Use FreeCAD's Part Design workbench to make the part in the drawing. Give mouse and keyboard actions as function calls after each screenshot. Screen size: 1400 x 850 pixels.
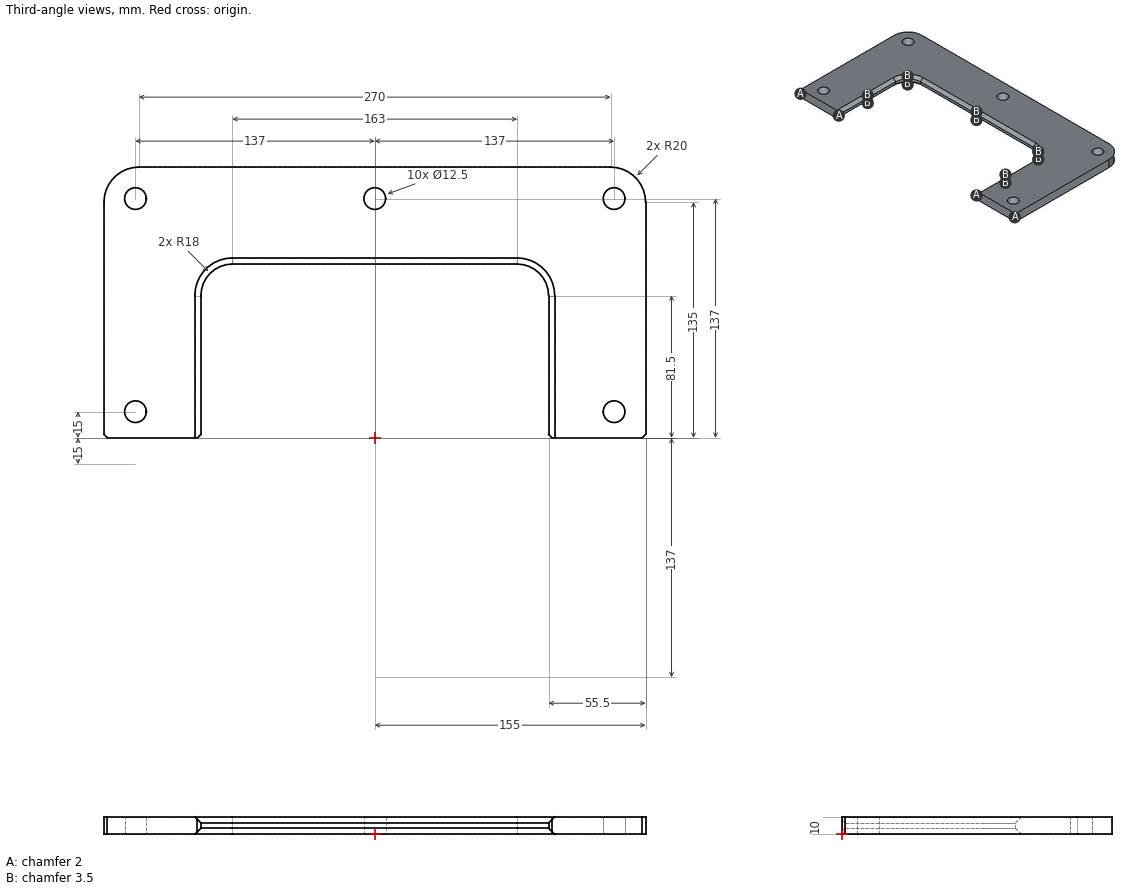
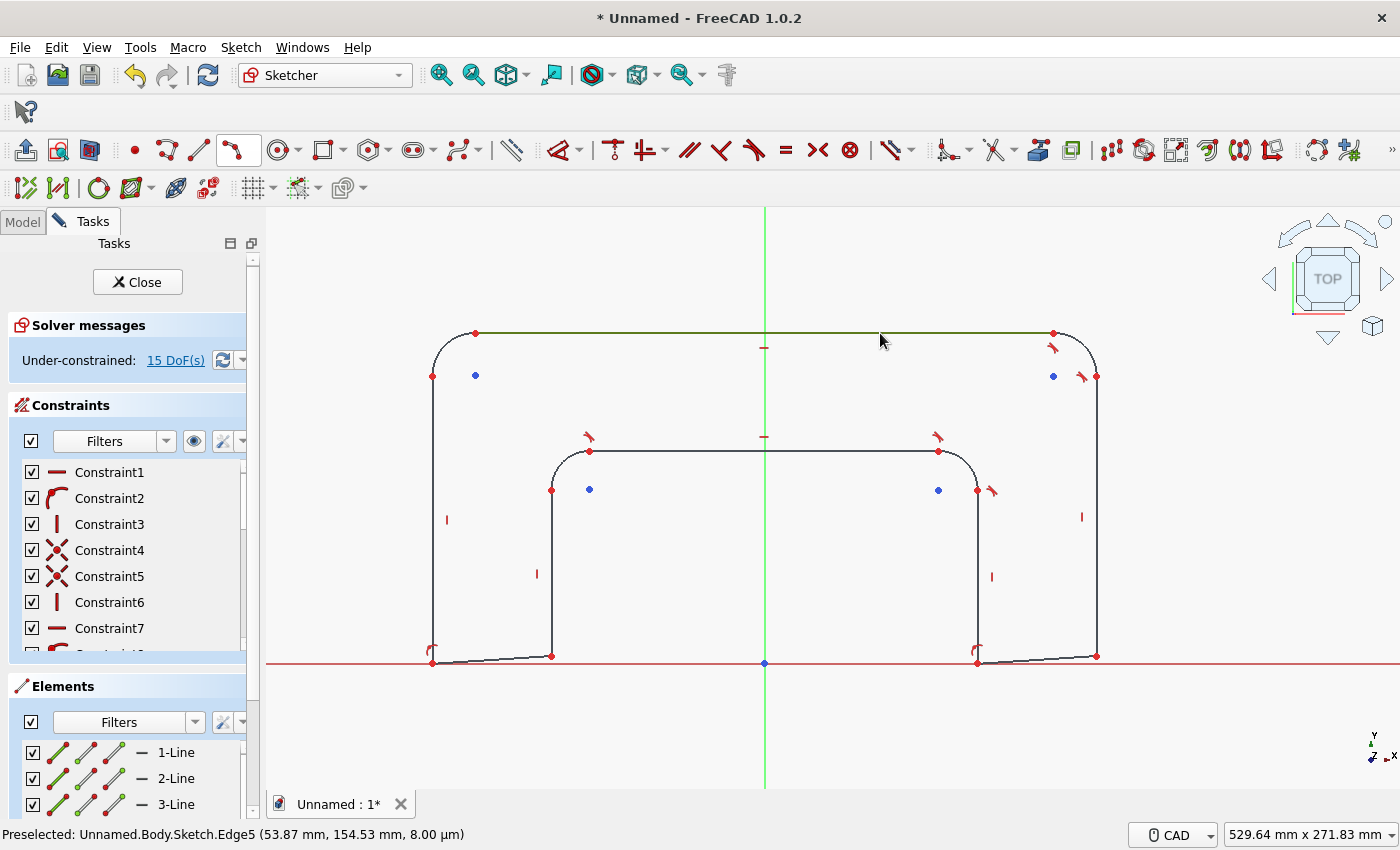
click(456, 337)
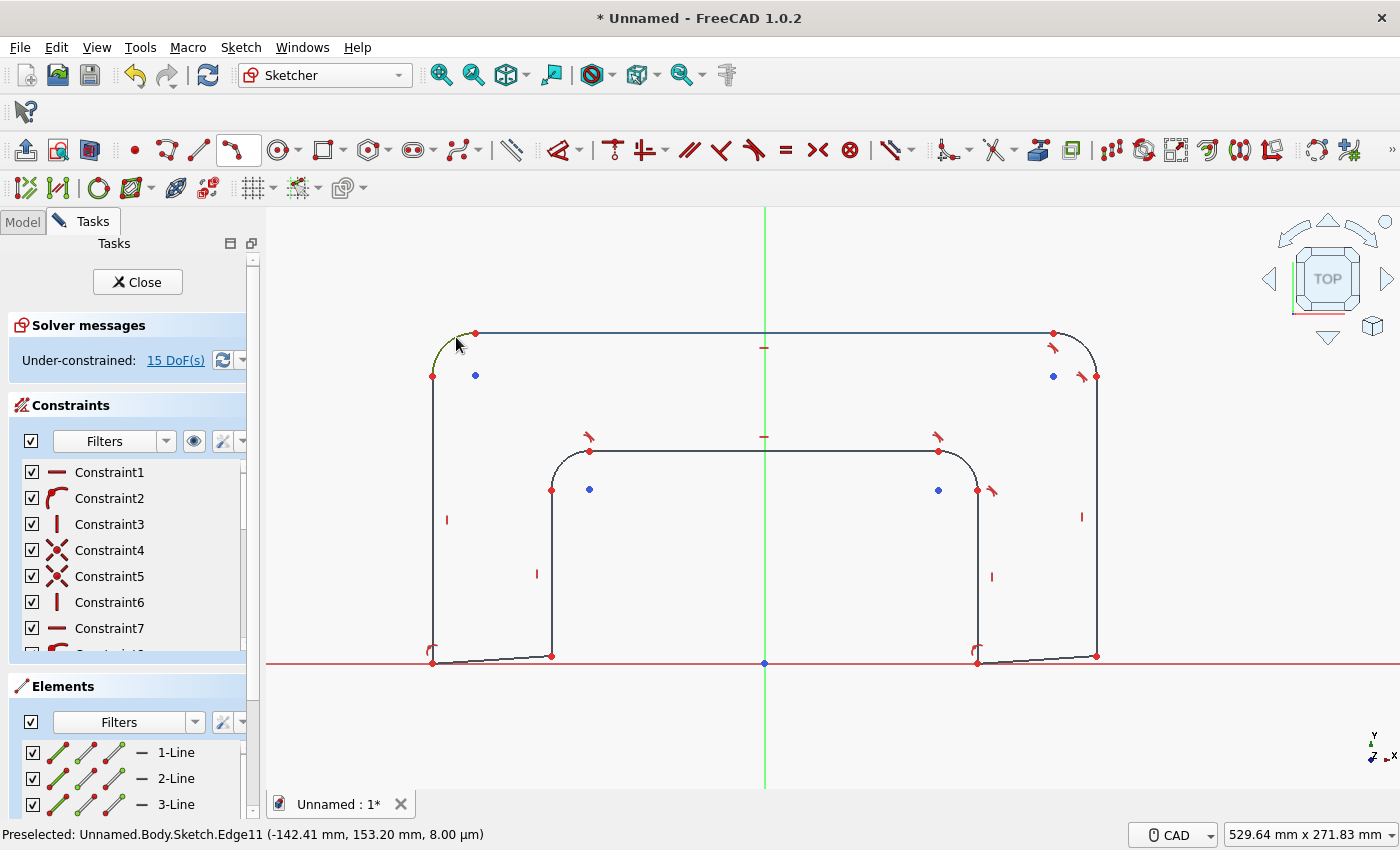
key(t)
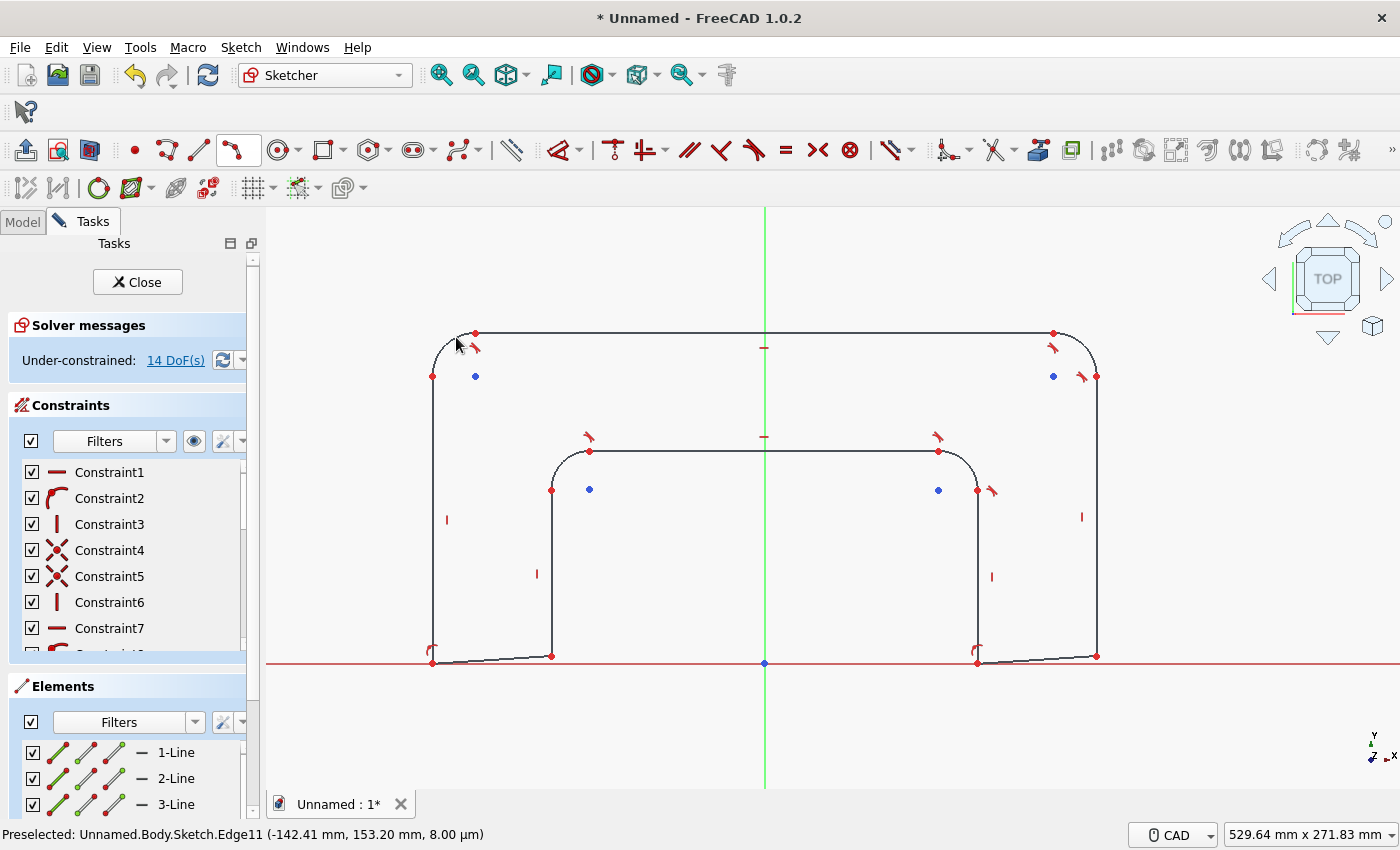
click(433, 462)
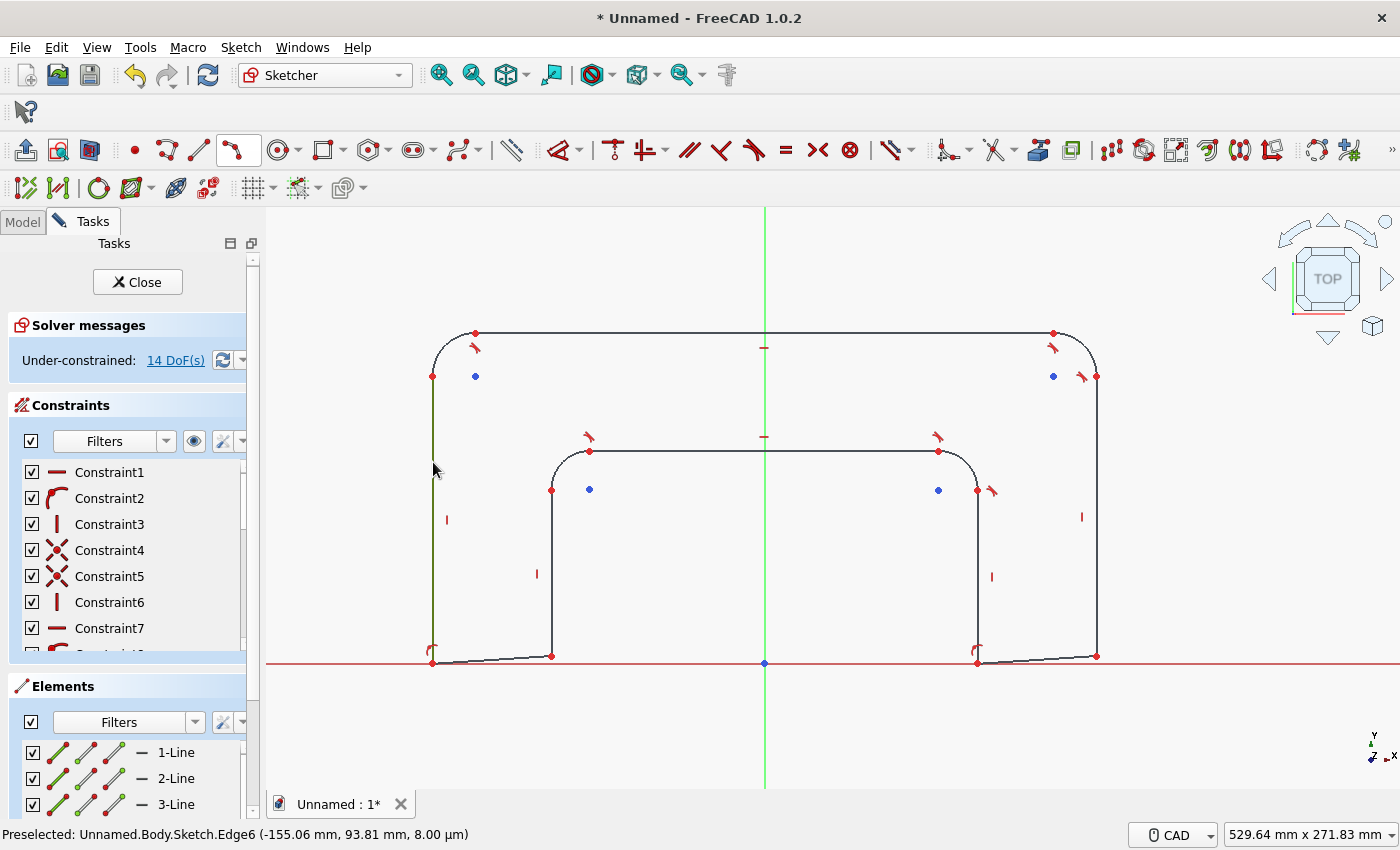
click(456, 338)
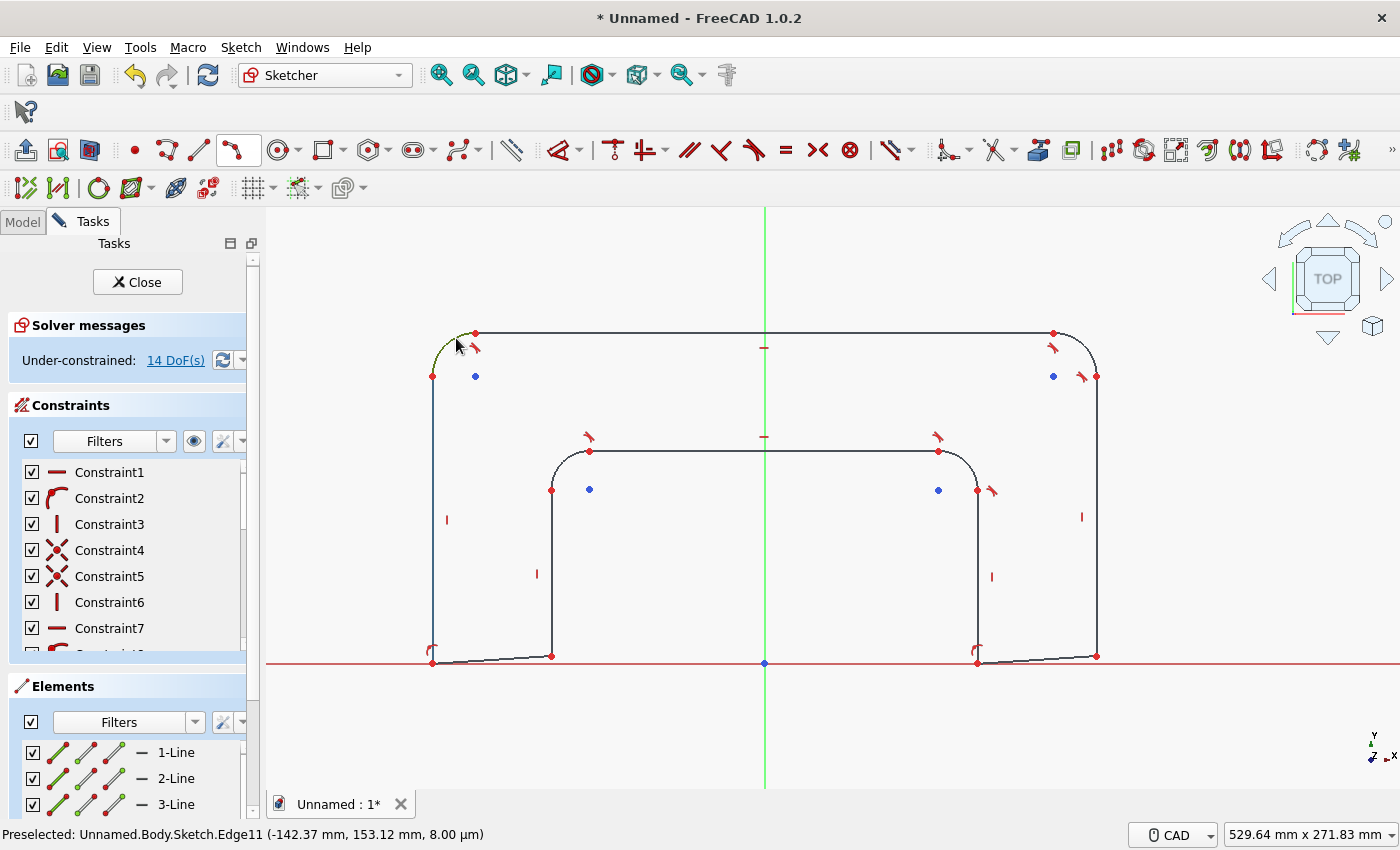
key(t)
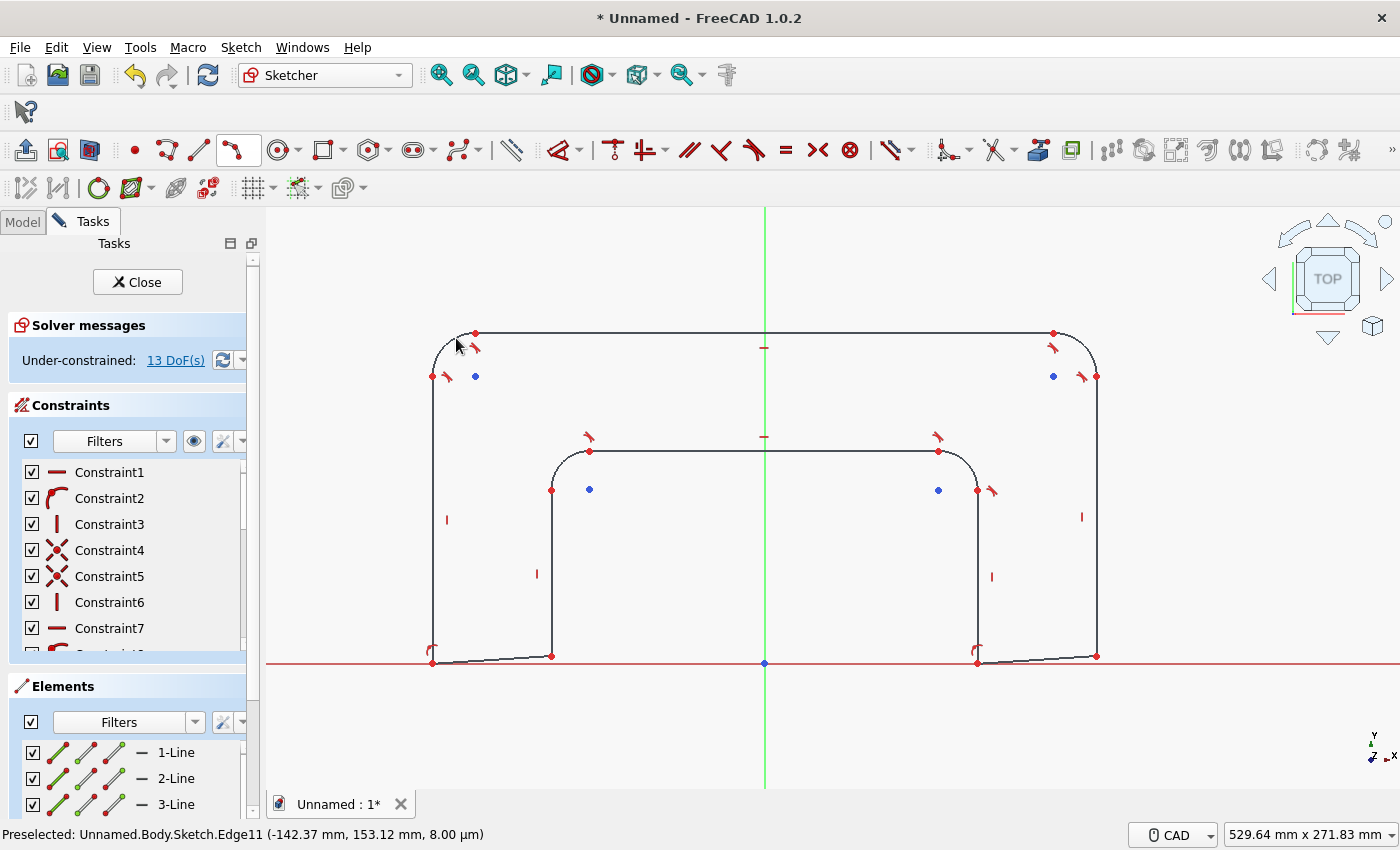
click(552, 606)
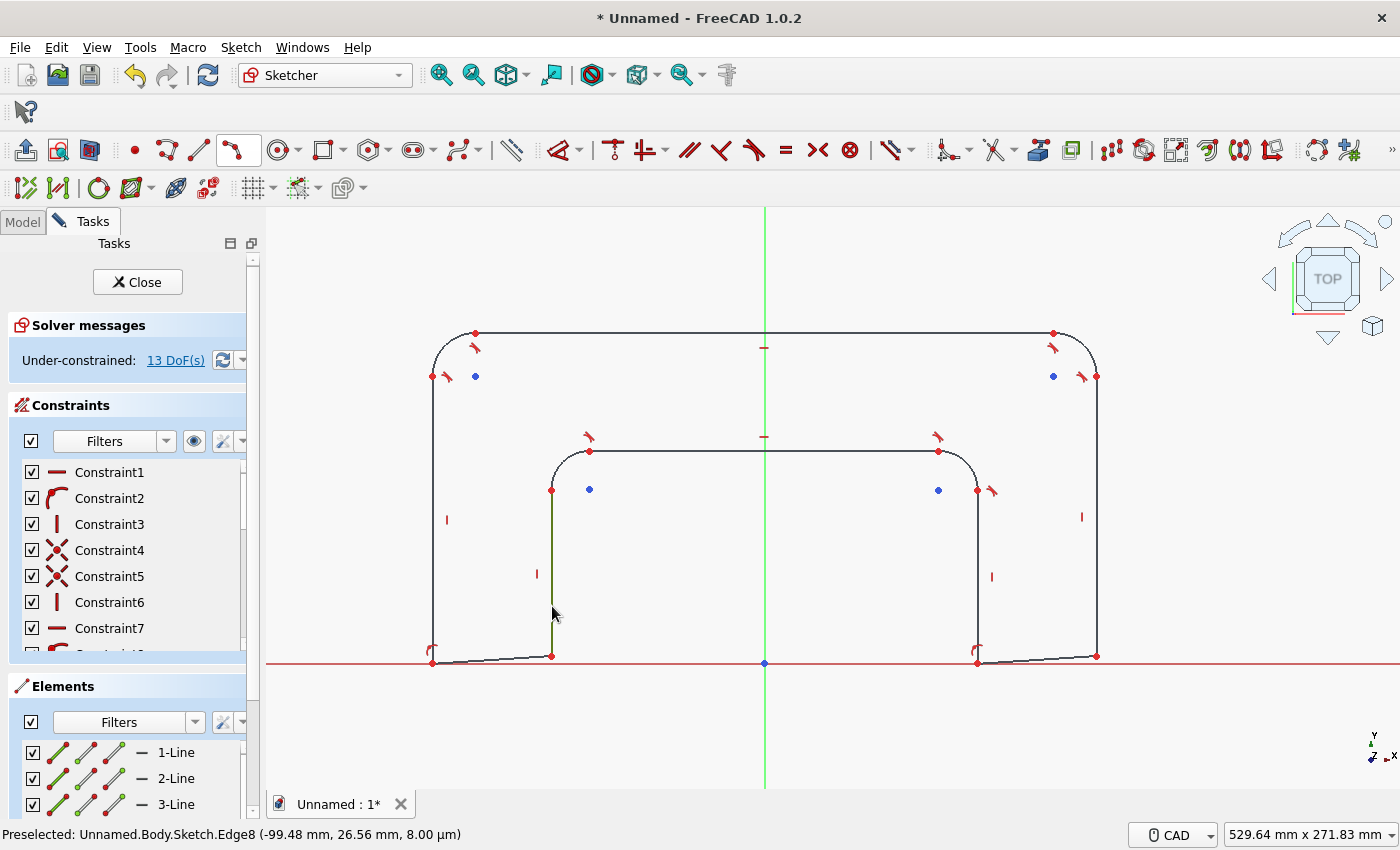
click(572, 455)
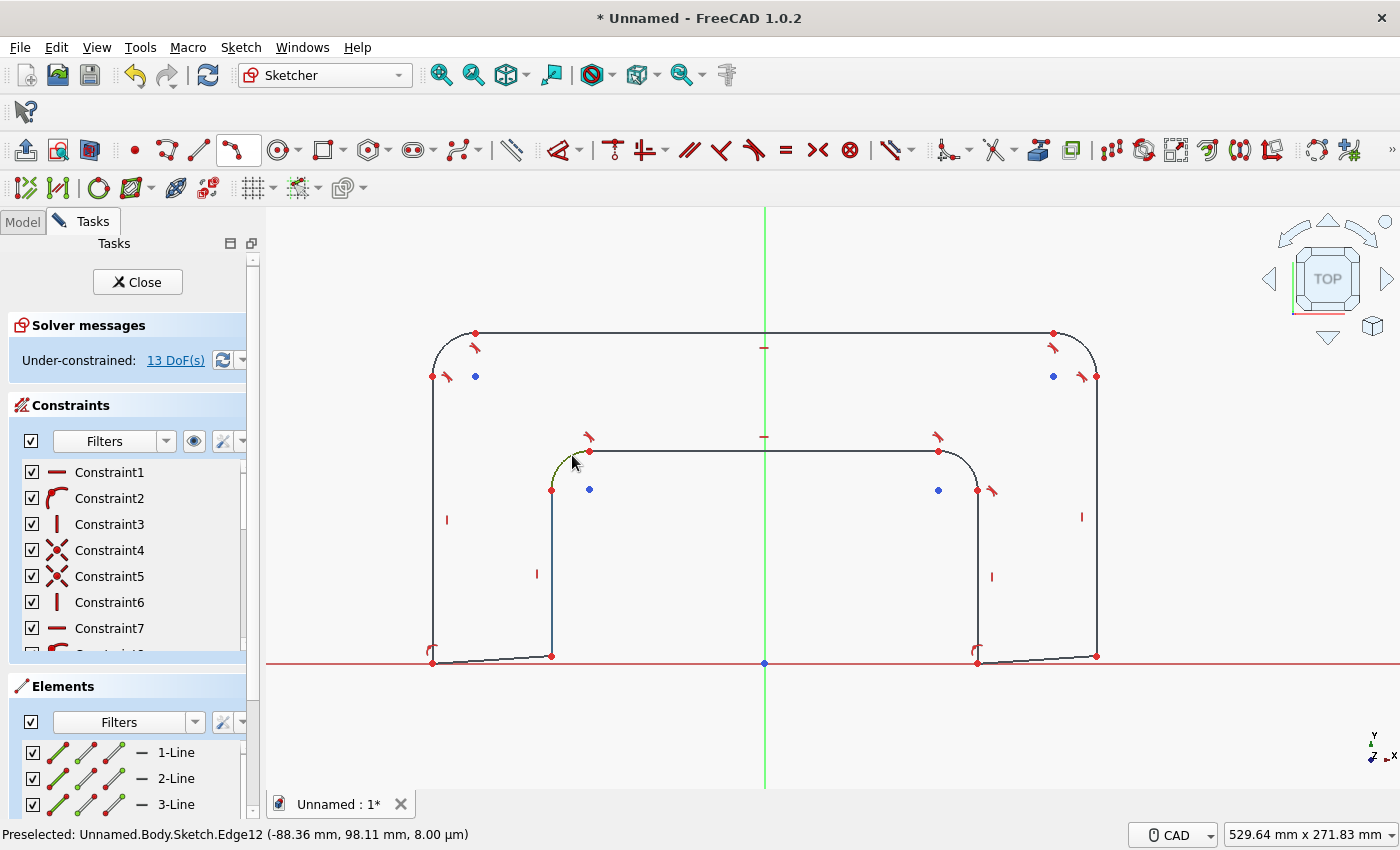
key(t)